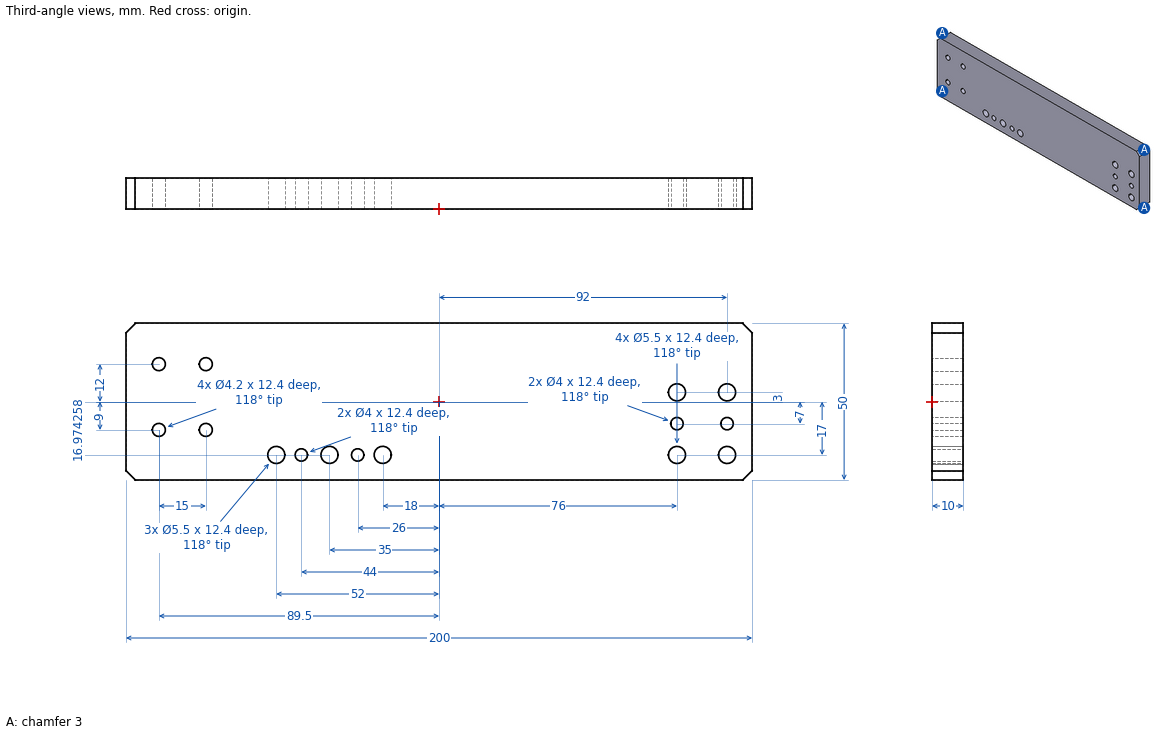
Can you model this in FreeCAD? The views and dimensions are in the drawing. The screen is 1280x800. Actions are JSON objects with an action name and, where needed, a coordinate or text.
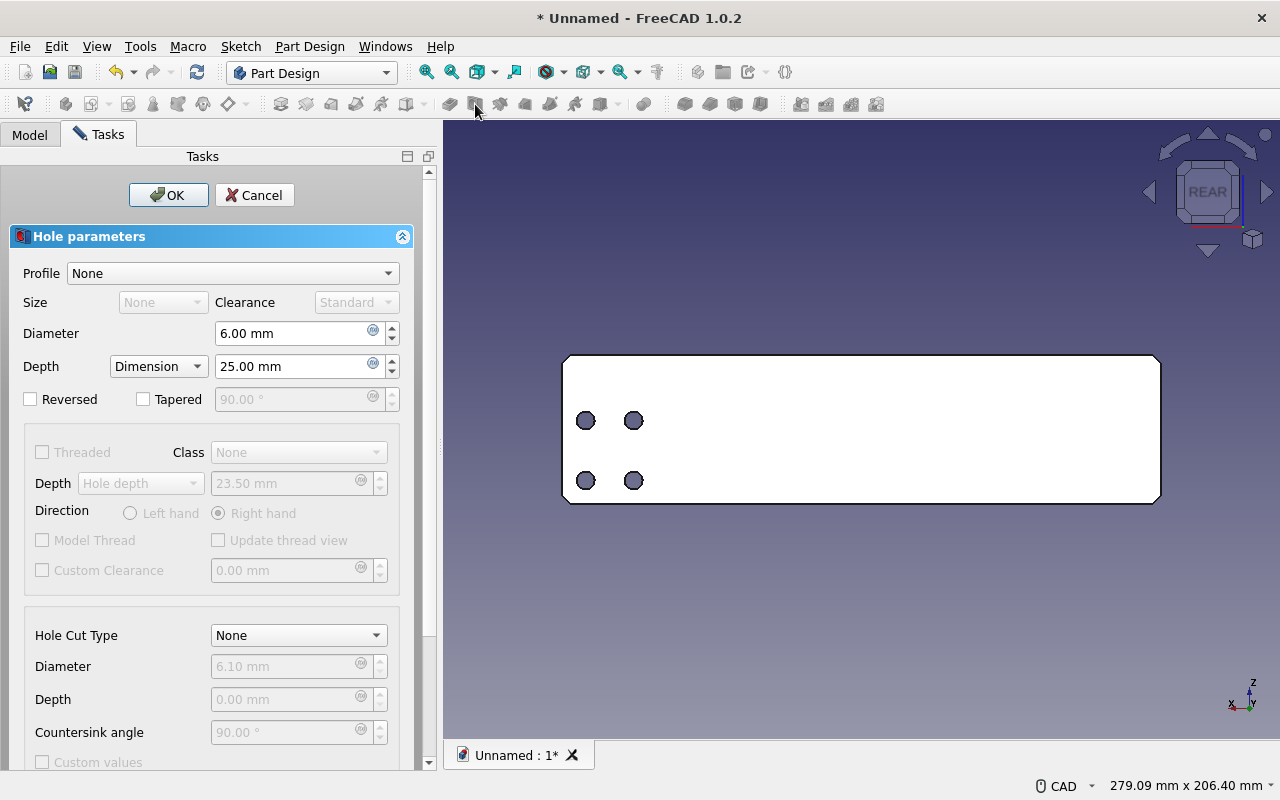
{"action": "triple_click", "coordinate": [300, 334]}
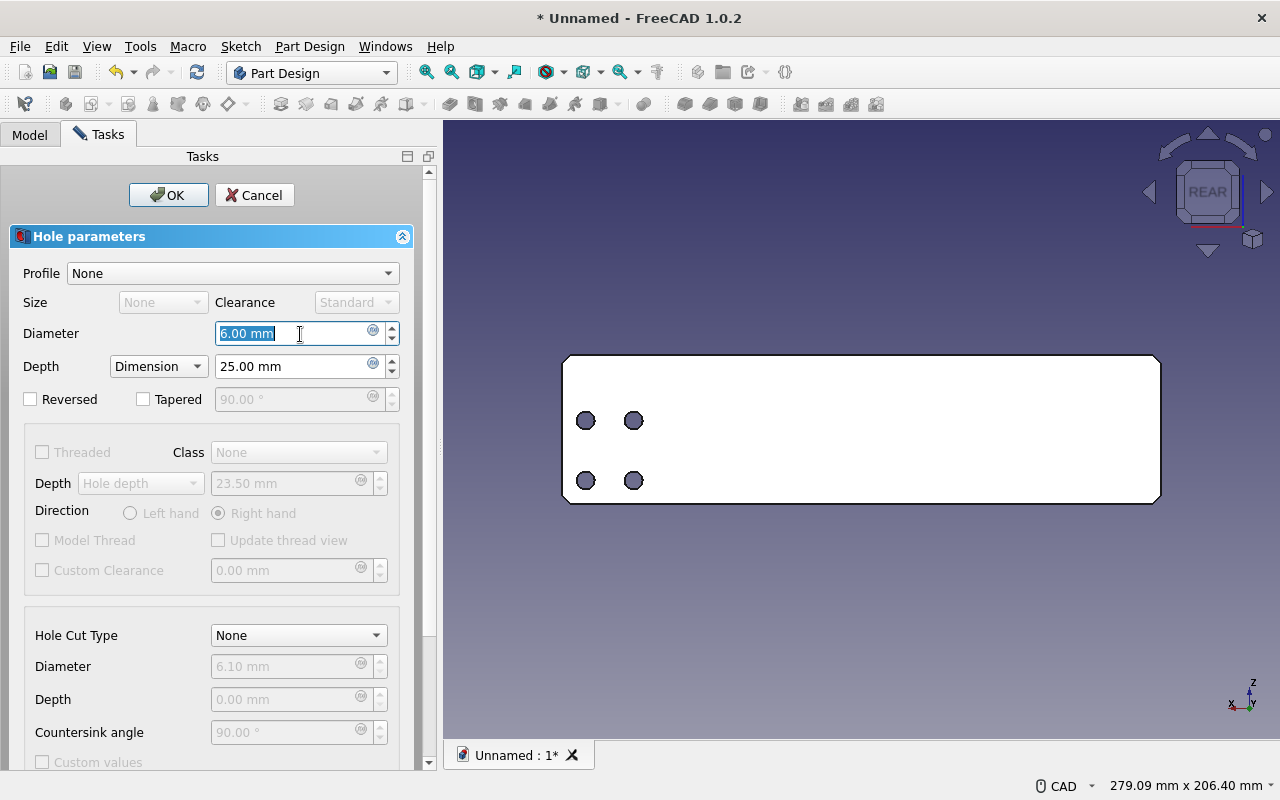
{"action": "type", "text": "5.5"}
{"action": "key", "text": "Tab"}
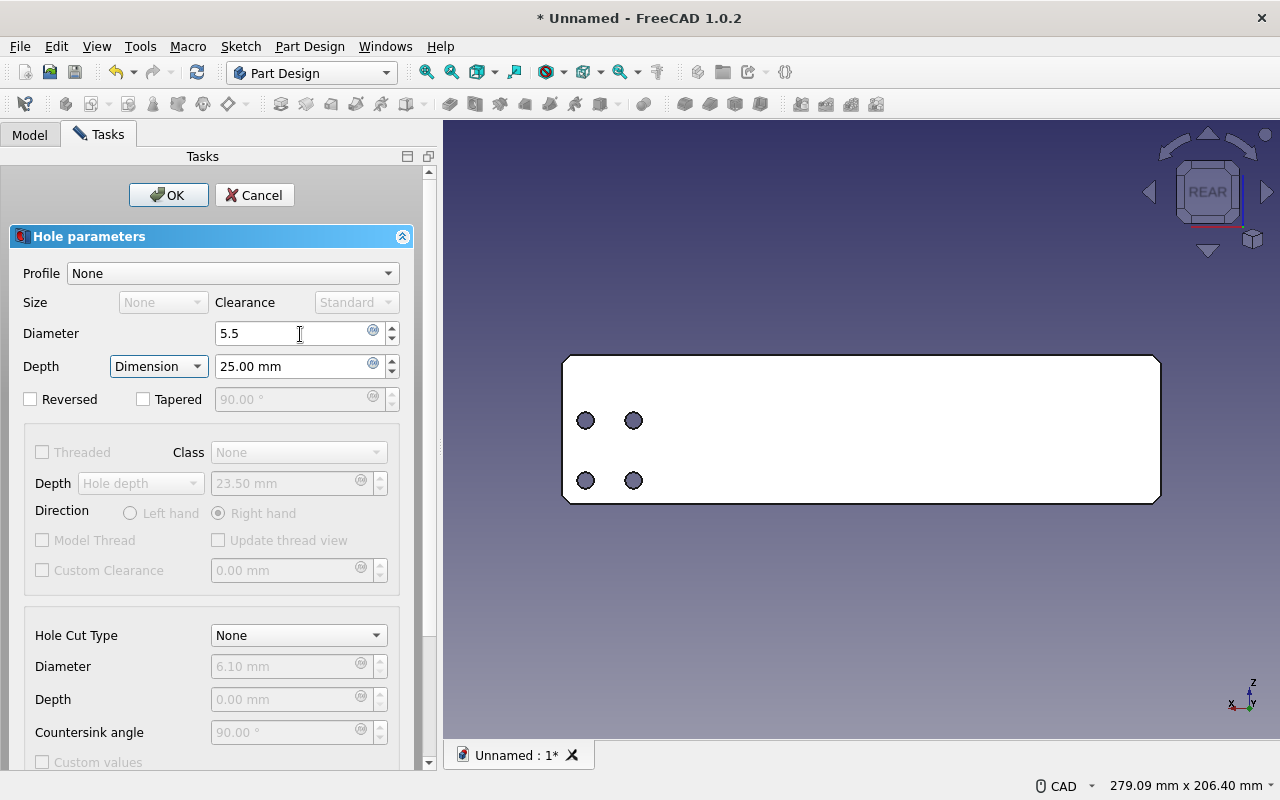
{"action": "triple_click", "coordinate": [300, 366]}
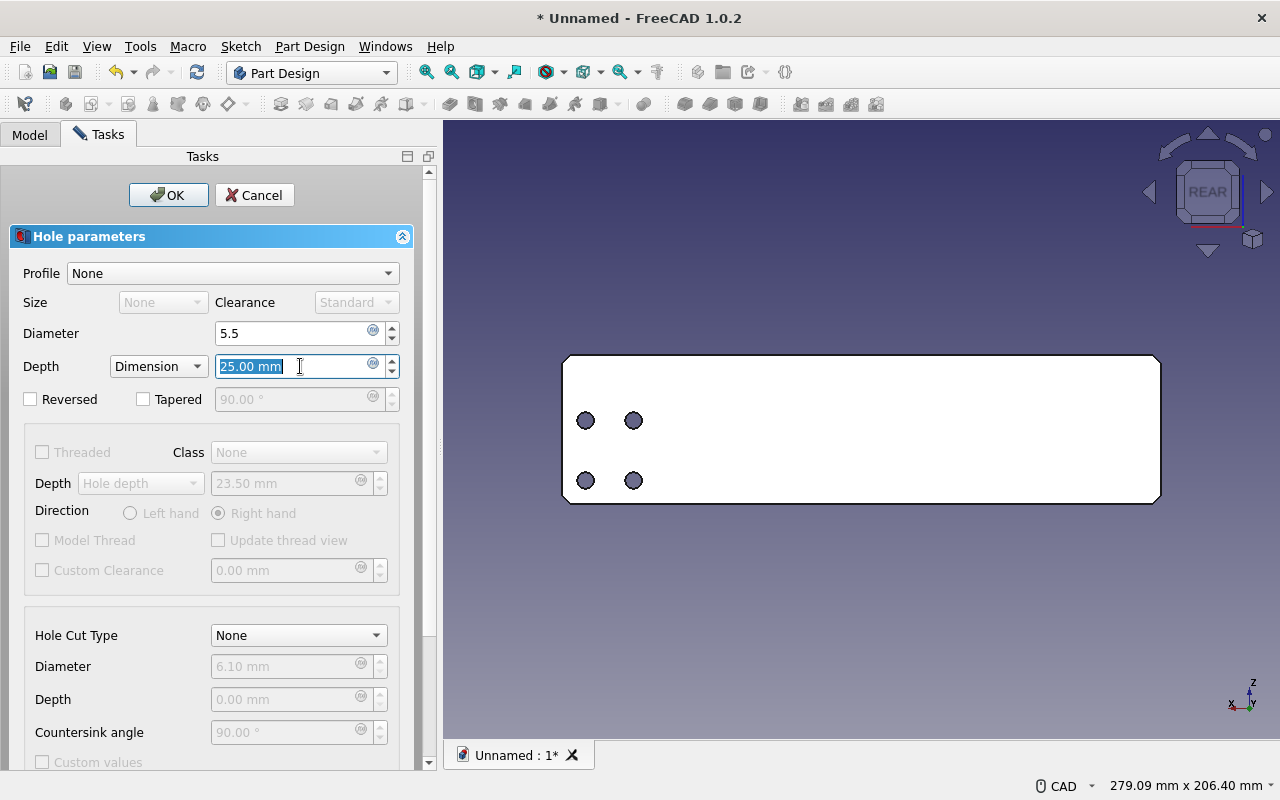
{"action": "type", "text": "12.4"}
{"action": "key", "text": "Tab"}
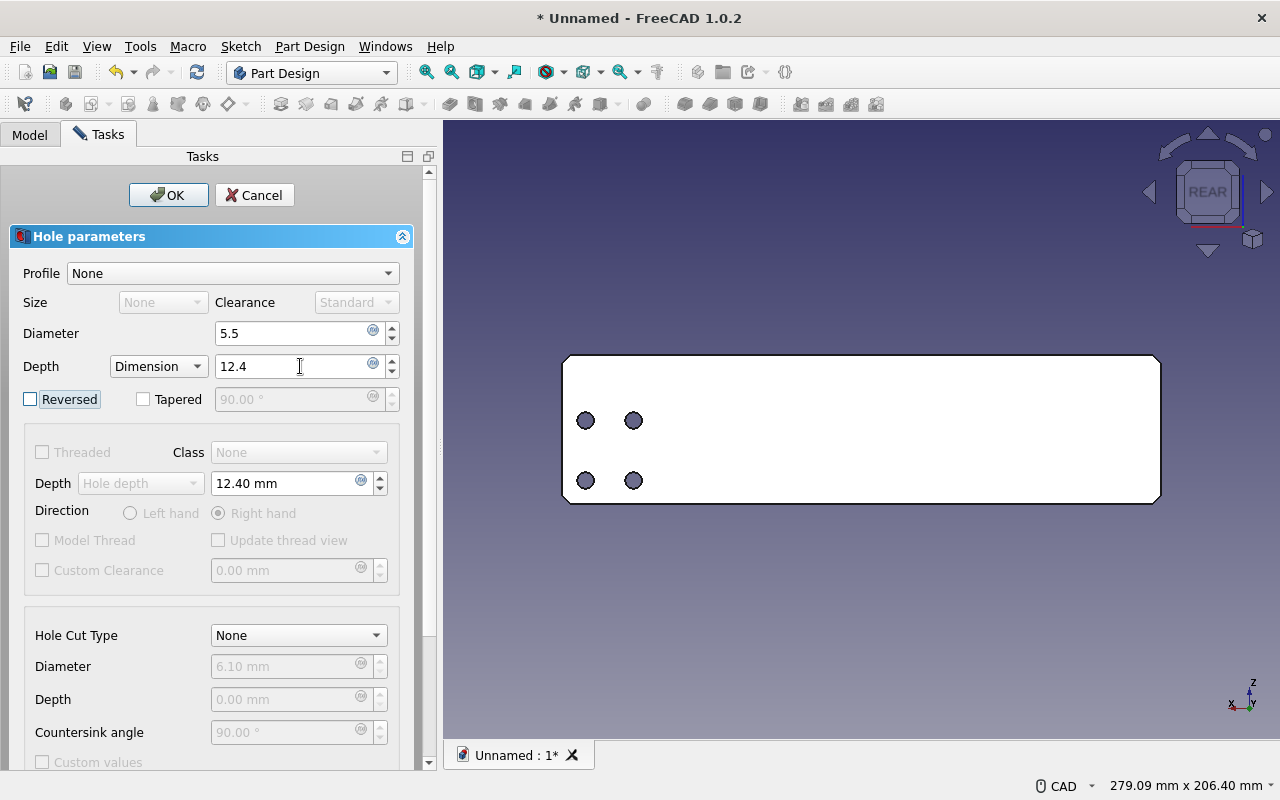
{"action": "left_click", "coordinate": [169, 195]}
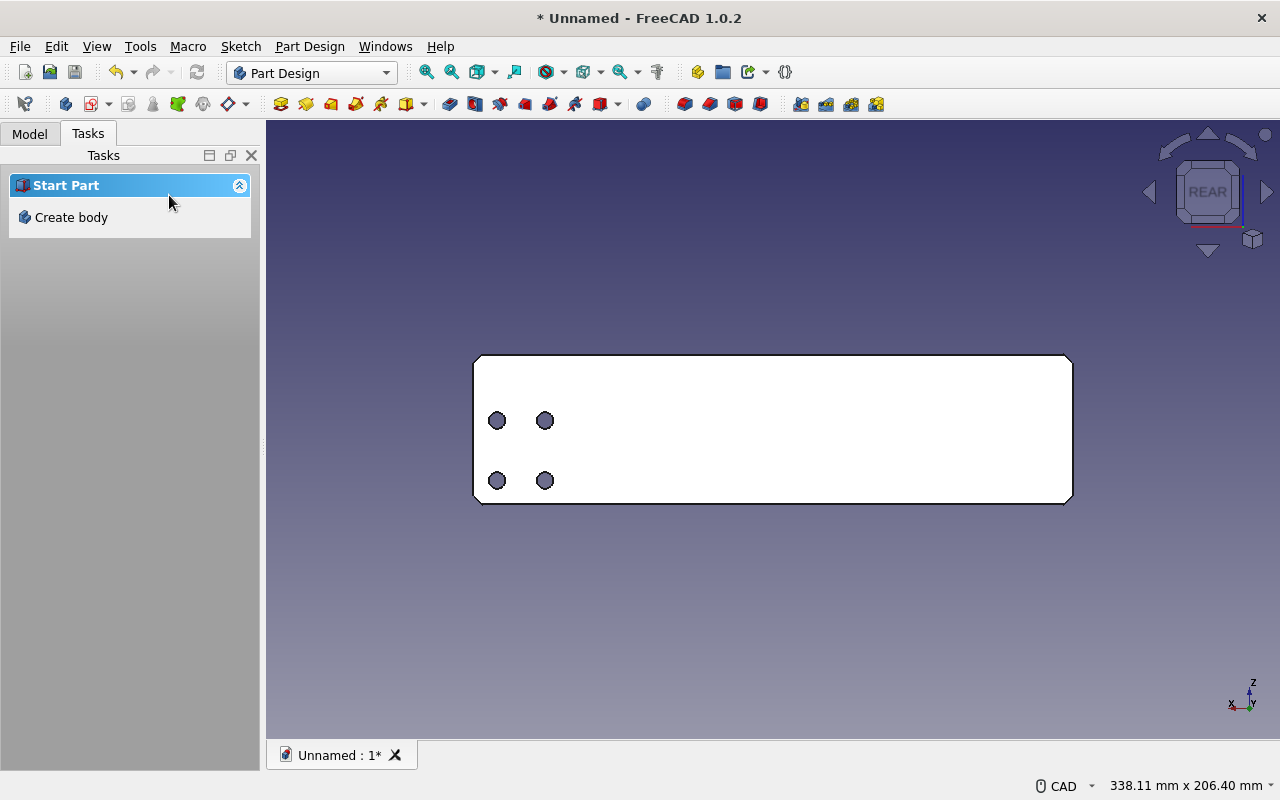
{"action": "left_click", "coordinate": [687, 429]}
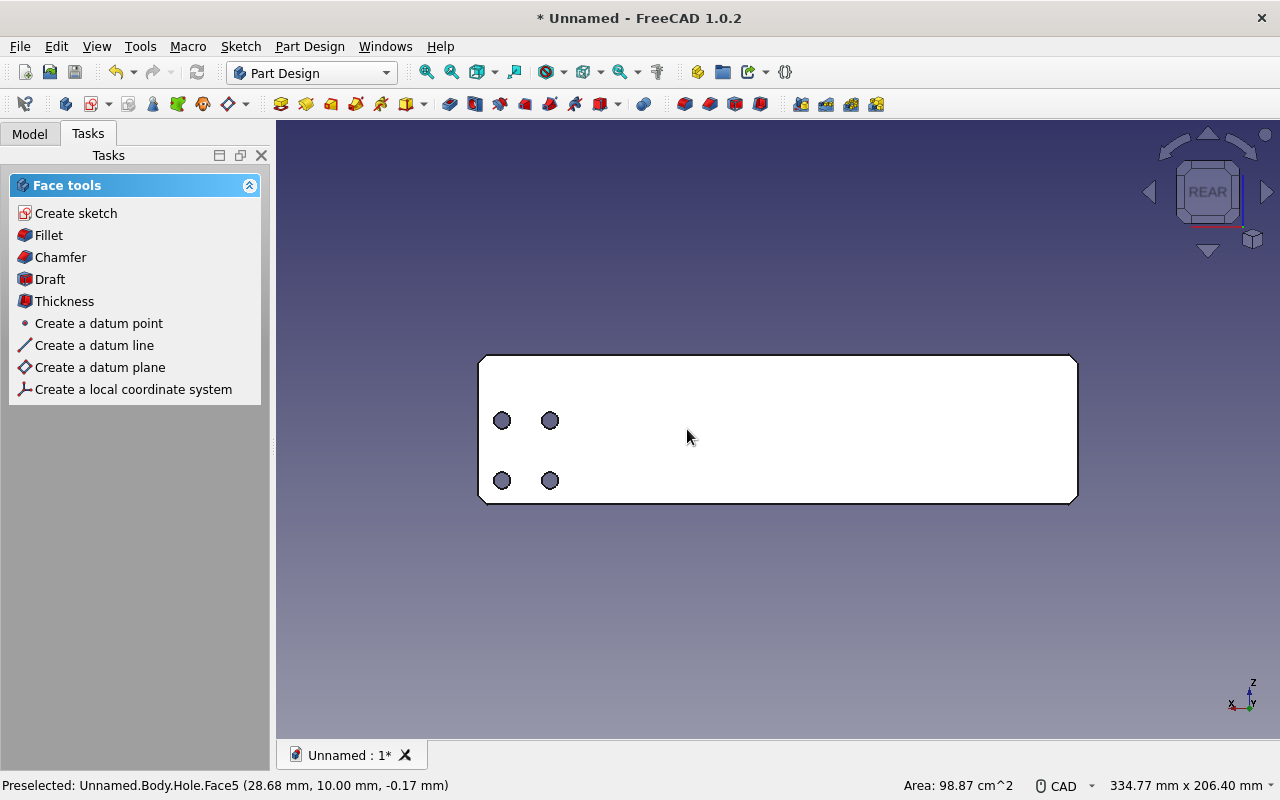
{"action": "left_click", "coordinate": [90, 104]}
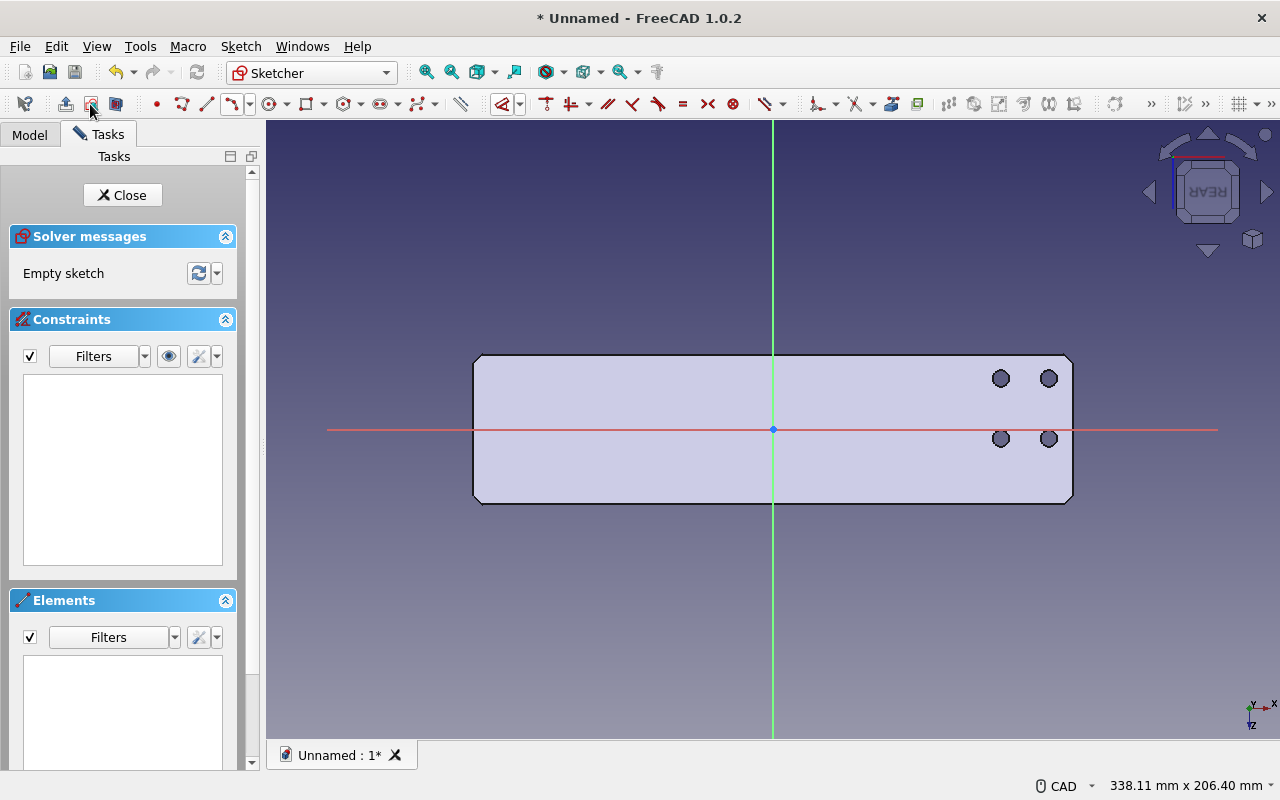
{"action": "scroll", "coordinate": [1065, 406], "scroll_direction": "up", "scroll_amount": 11}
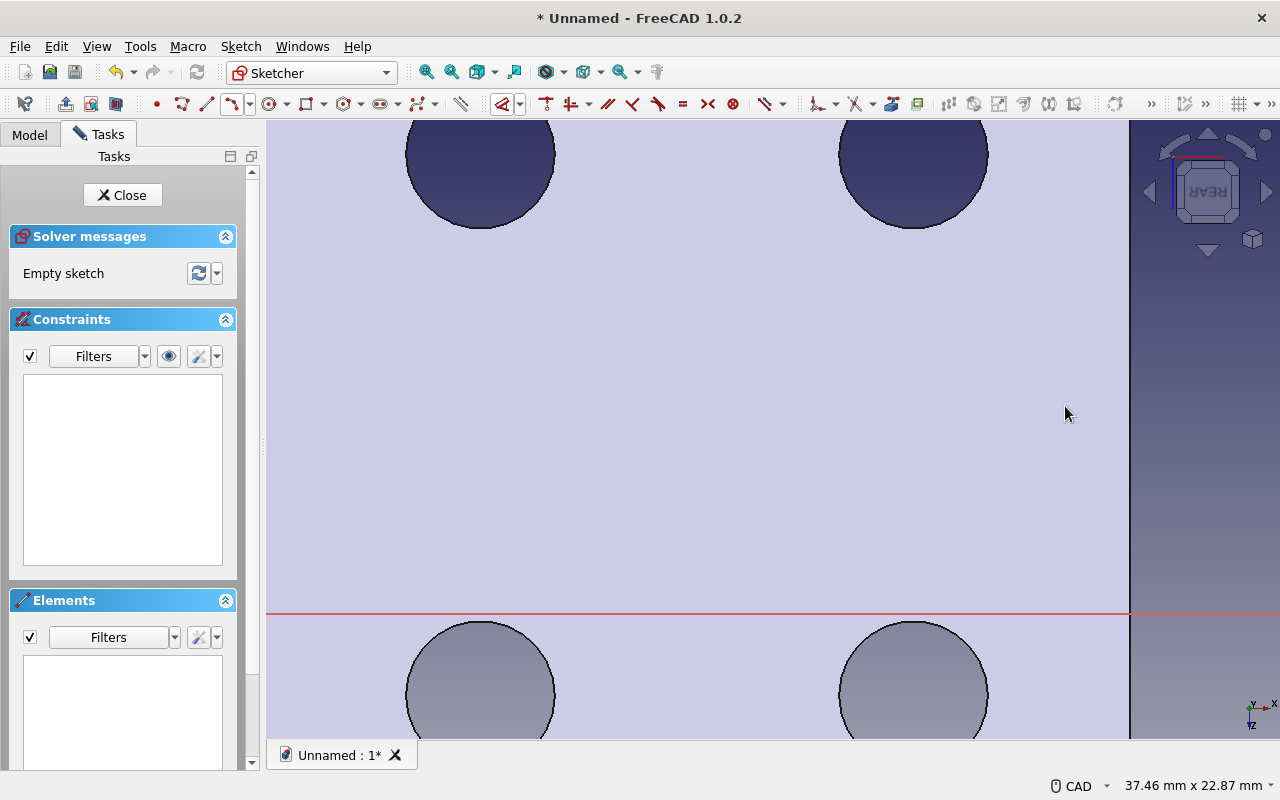
{"action": "key", "text": "g c"}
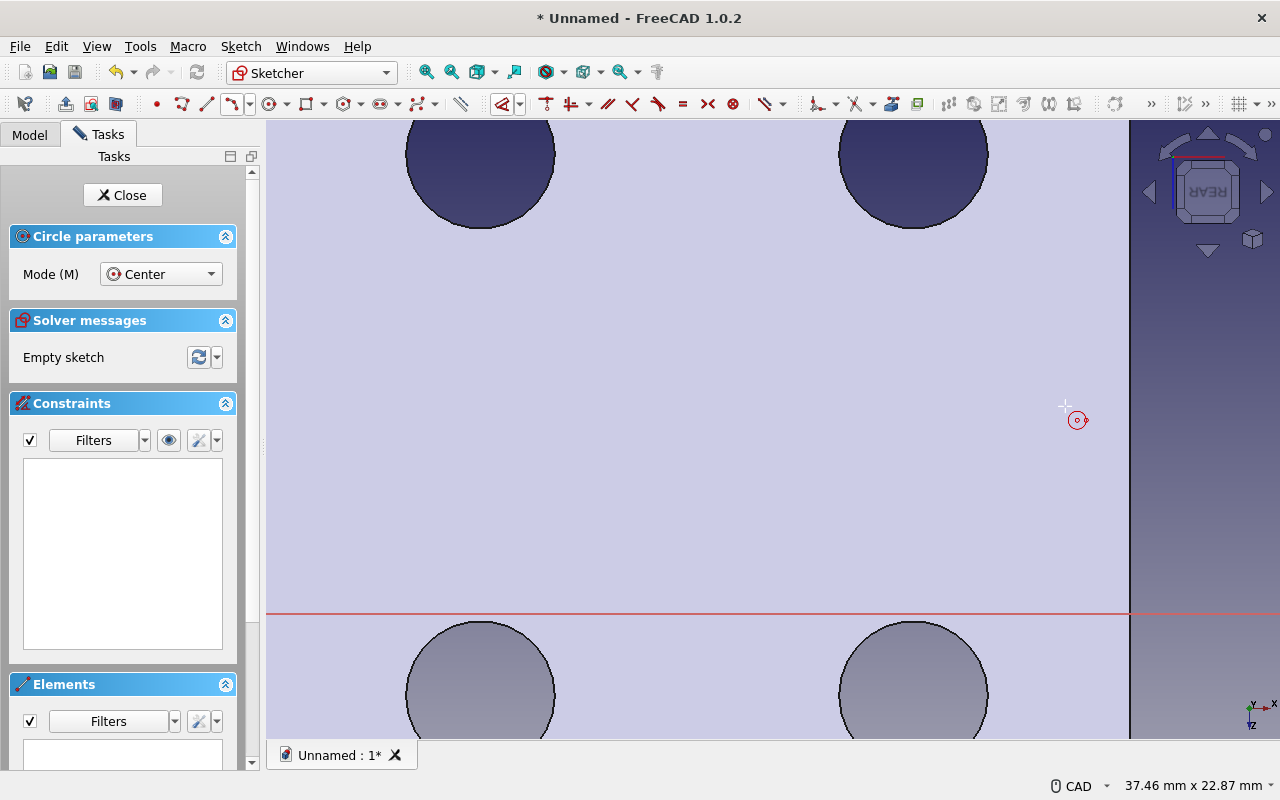
{"action": "left_click", "coordinate": [480, 425]}
{"action": "left_click", "coordinate": [519, 387]}